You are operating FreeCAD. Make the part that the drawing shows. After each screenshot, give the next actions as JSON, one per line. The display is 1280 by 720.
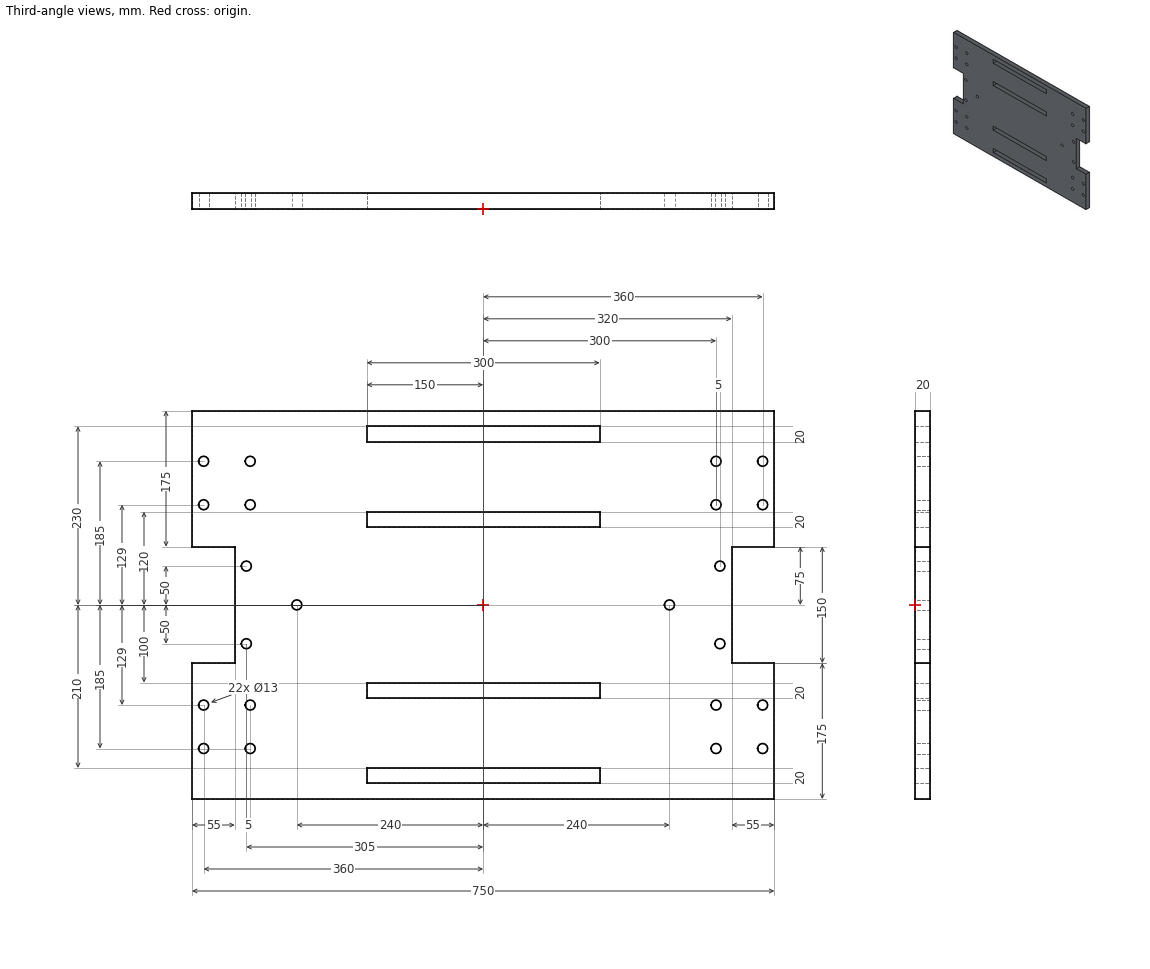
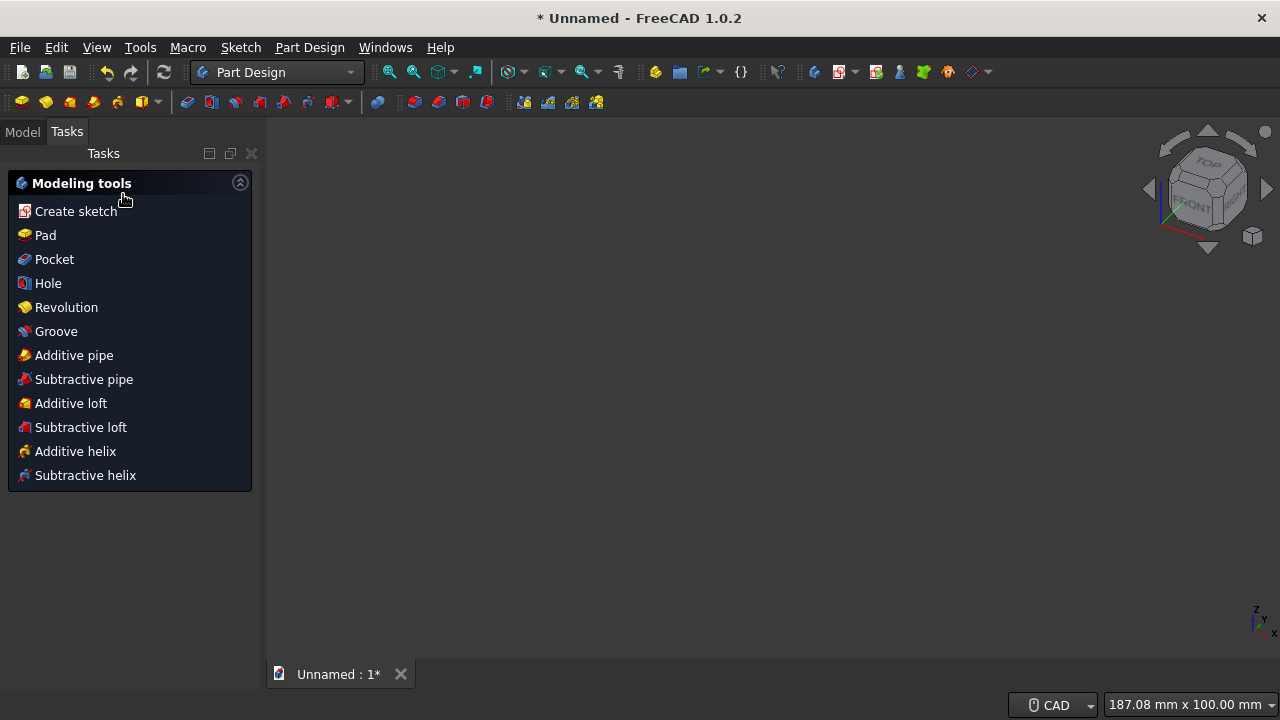
{"action": "left_click", "coordinate": [22, 102]}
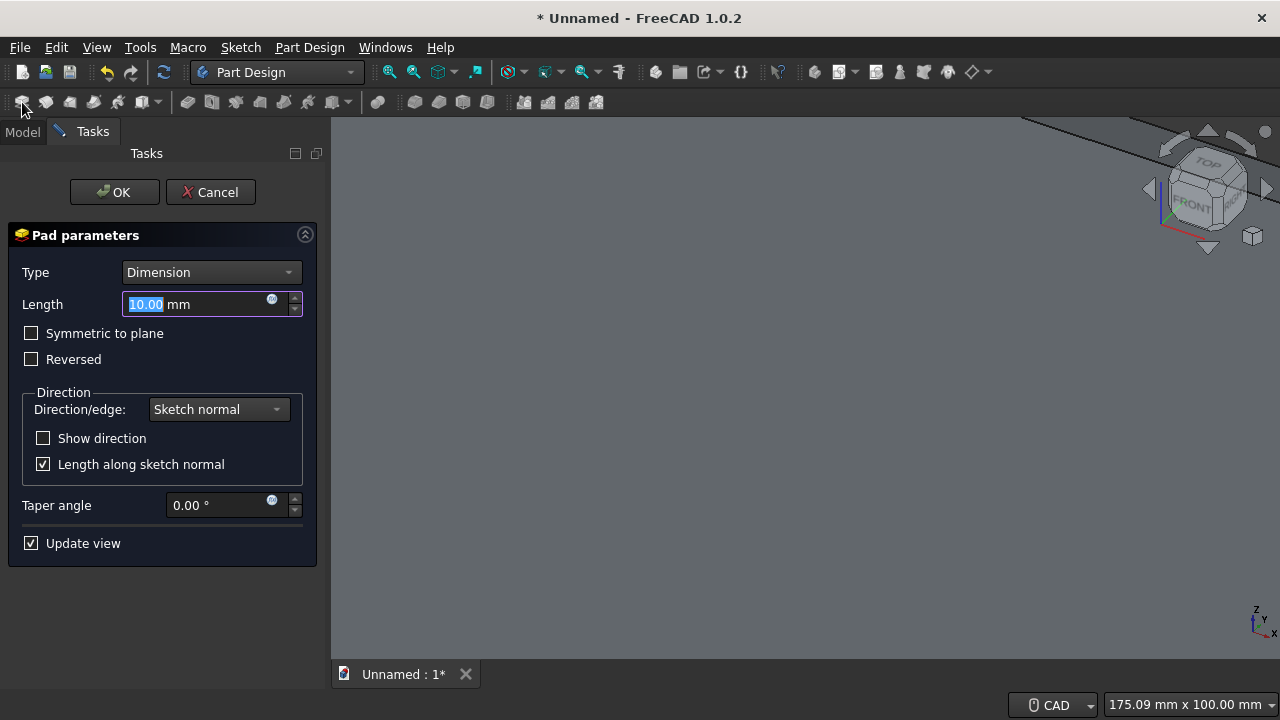
{"action": "type", "text": "20"}
{"action": "key", "text": "Tab"}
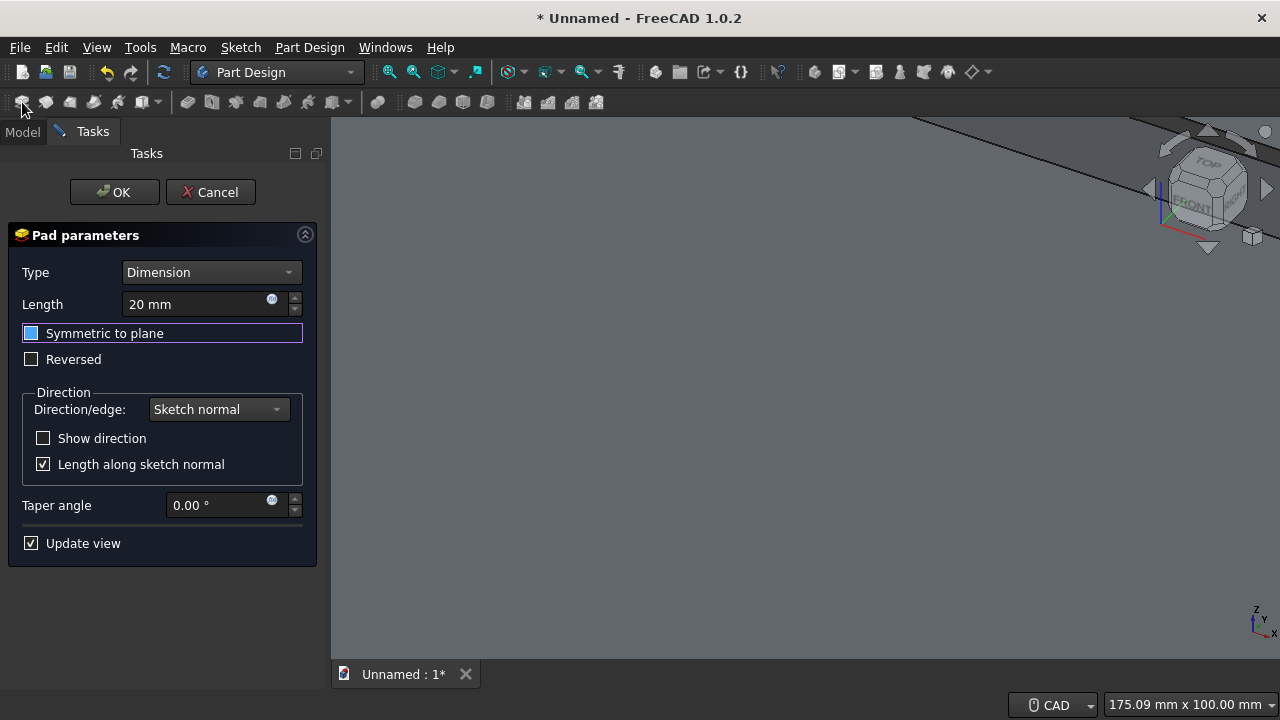
{"action": "left_click", "coordinate": [30, 359]}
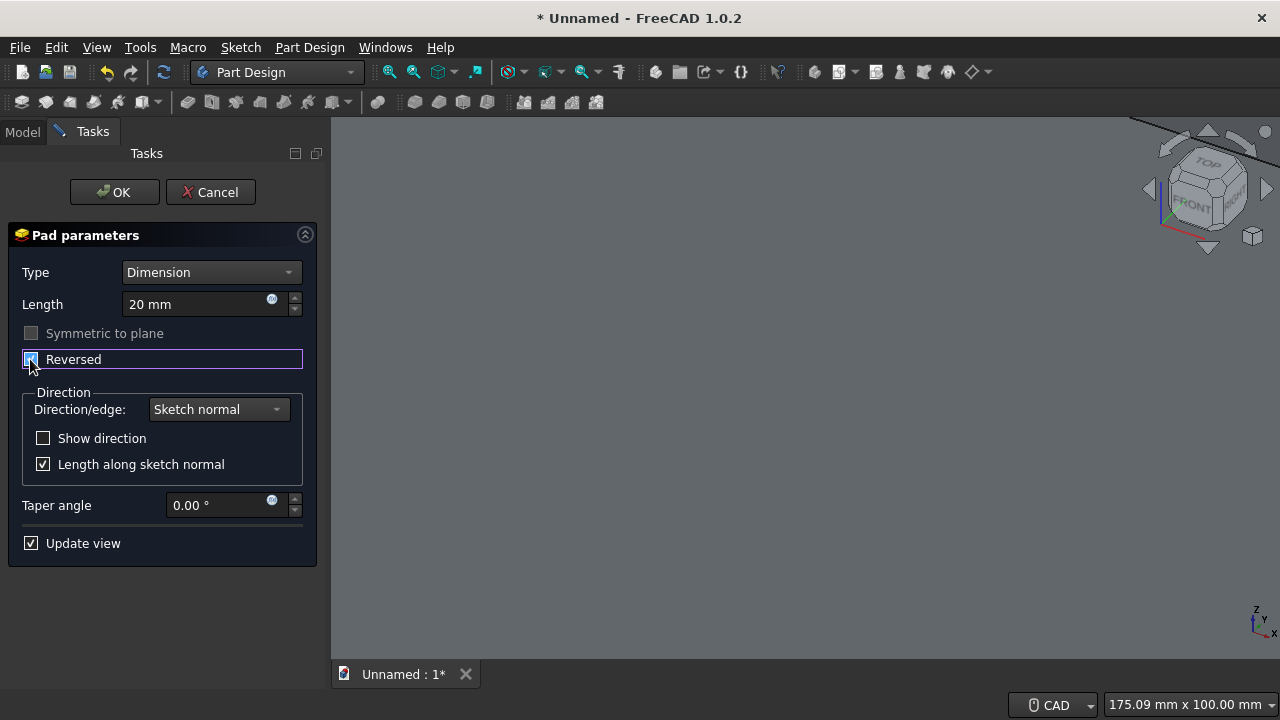
{"action": "left_click", "coordinate": [115, 192]}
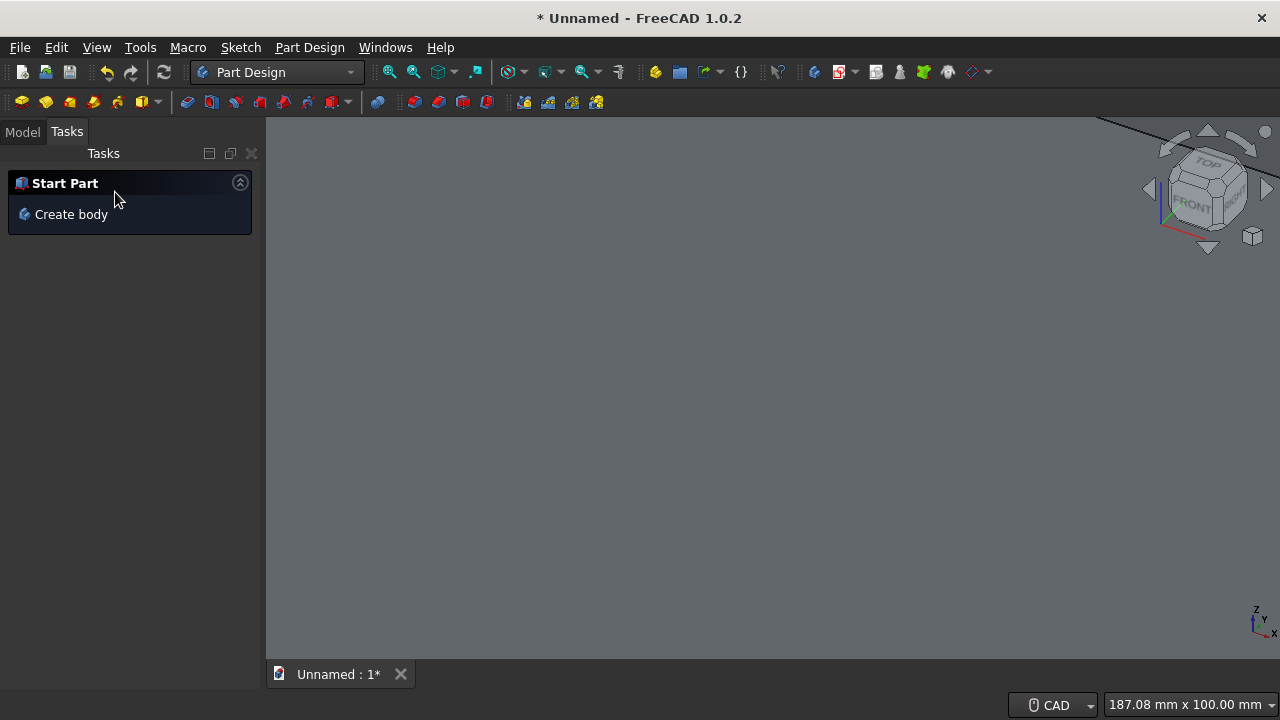
{"action": "left_click", "coordinate": [390, 72]}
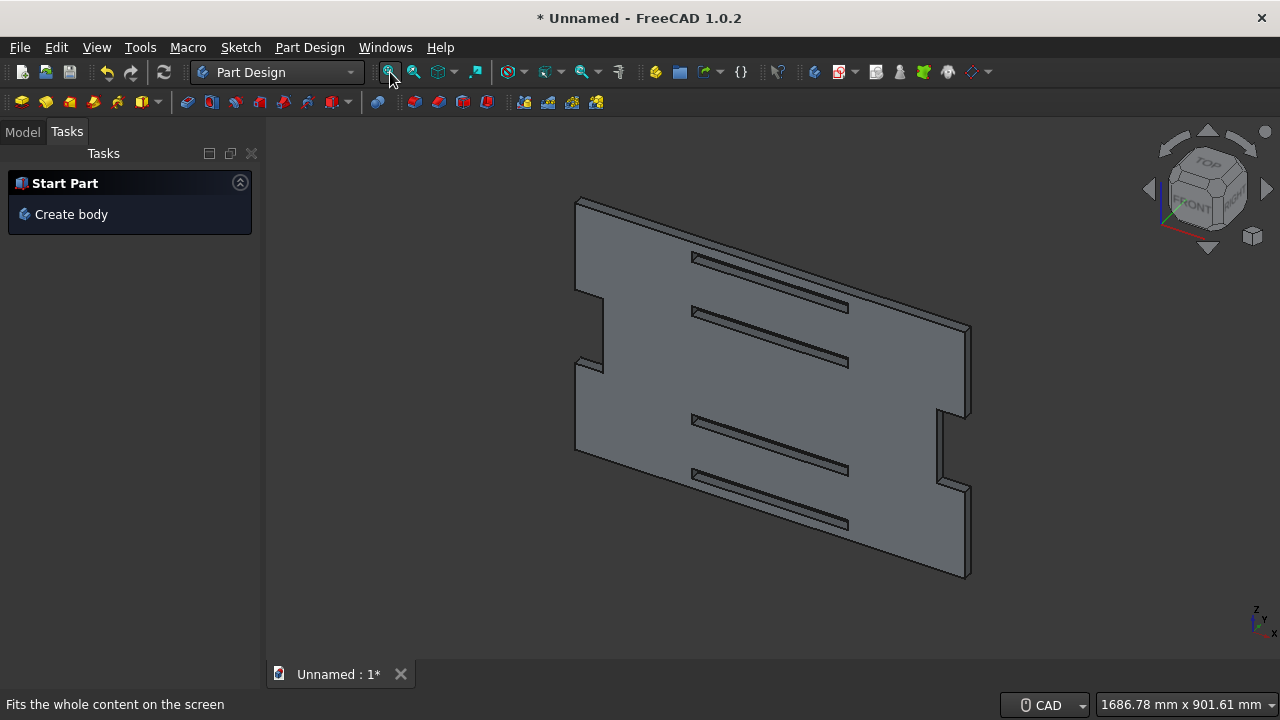
{"action": "key", "text": "4"}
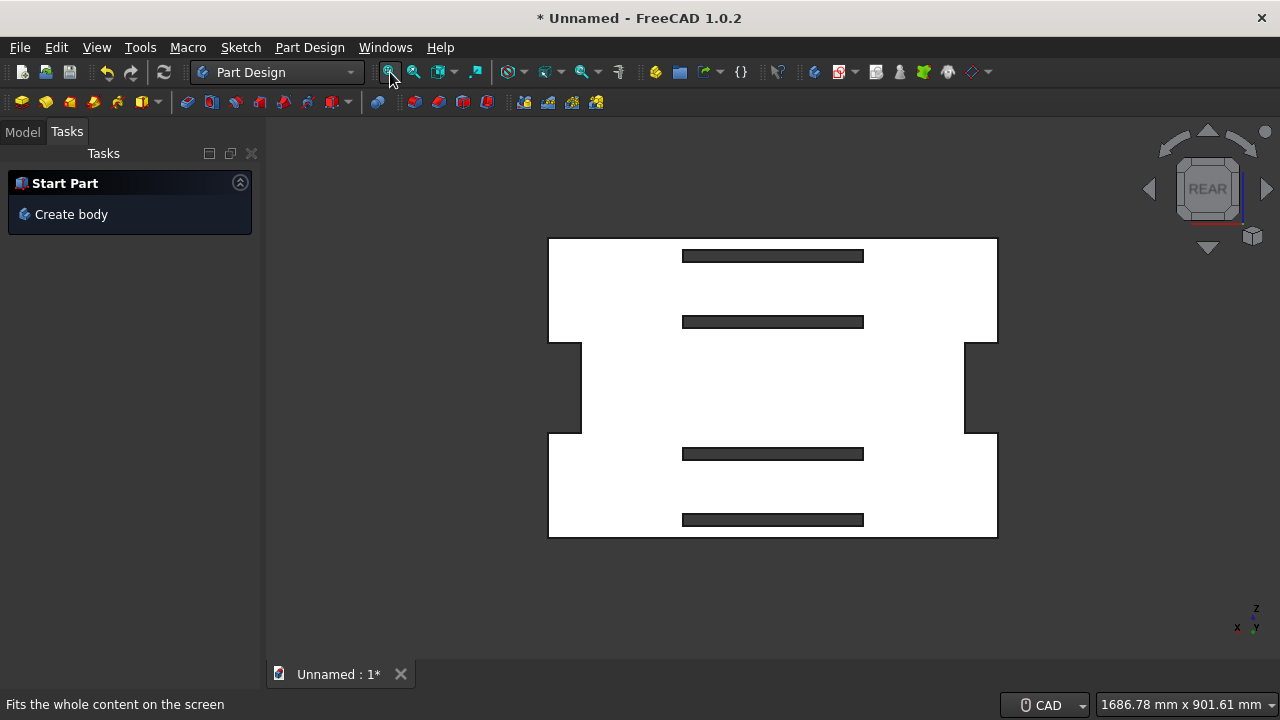
{"action": "left_click", "coordinate": [644, 387]}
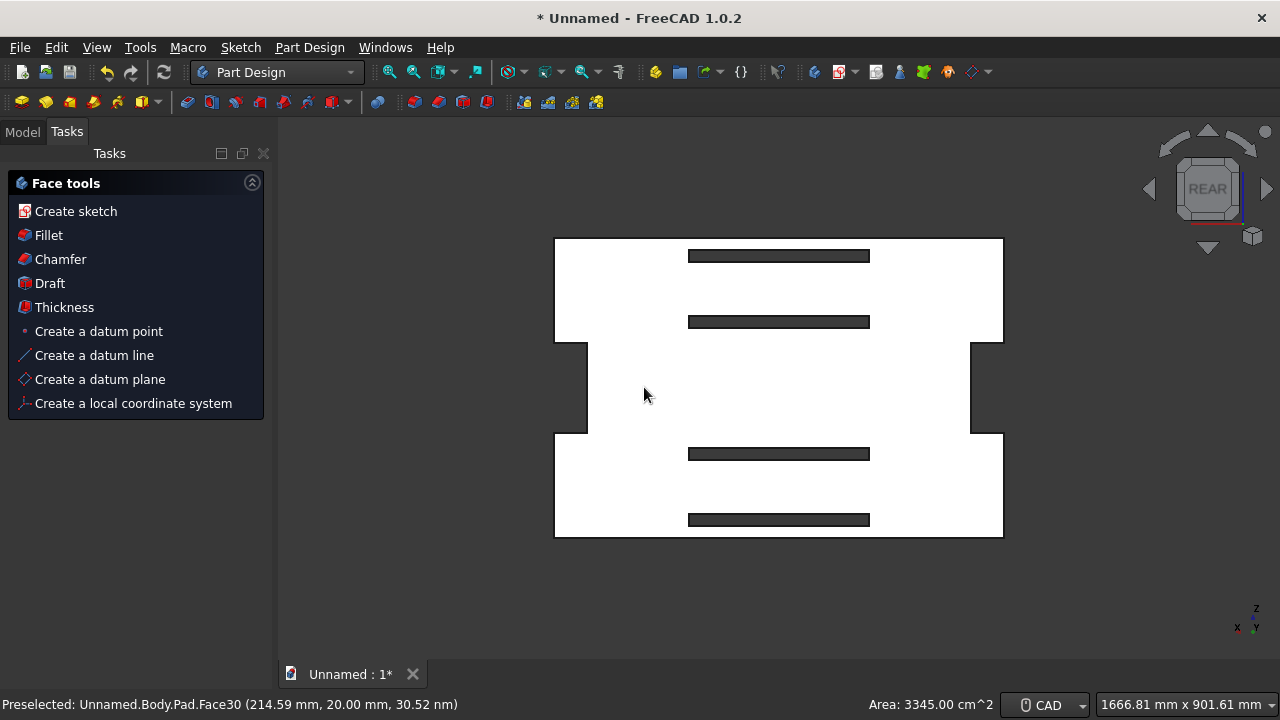
{"action": "left_click", "coordinate": [840, 72]}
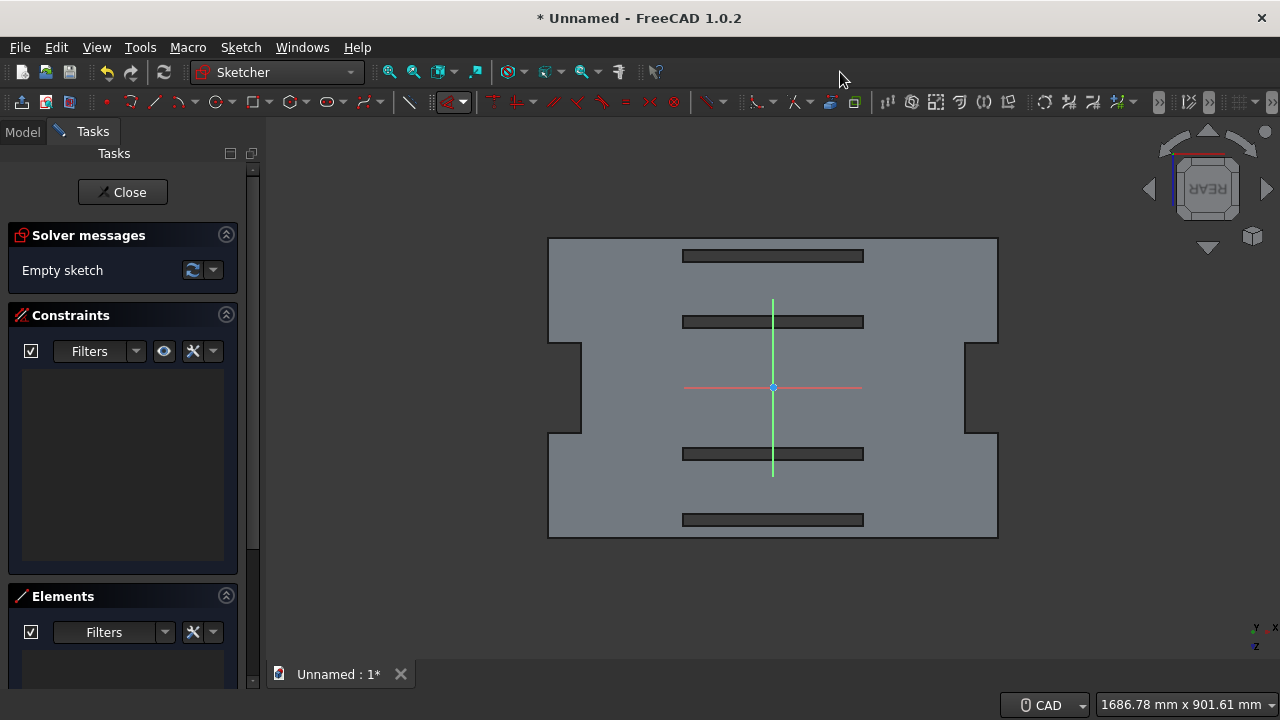
{"action": "left_click", "coordinate": [216, 102]}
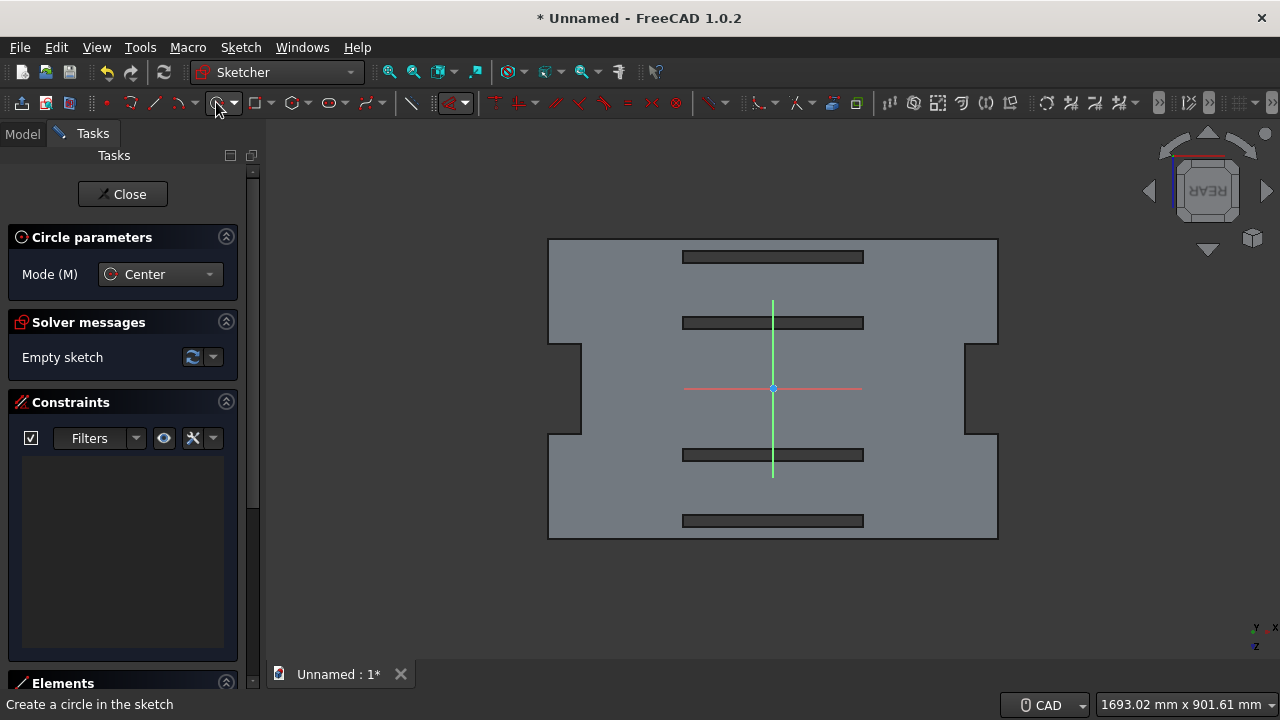
{"action": "scroll", "coordinate": [557, 312], "scroll_direction": "up", "scroll_amount": 9}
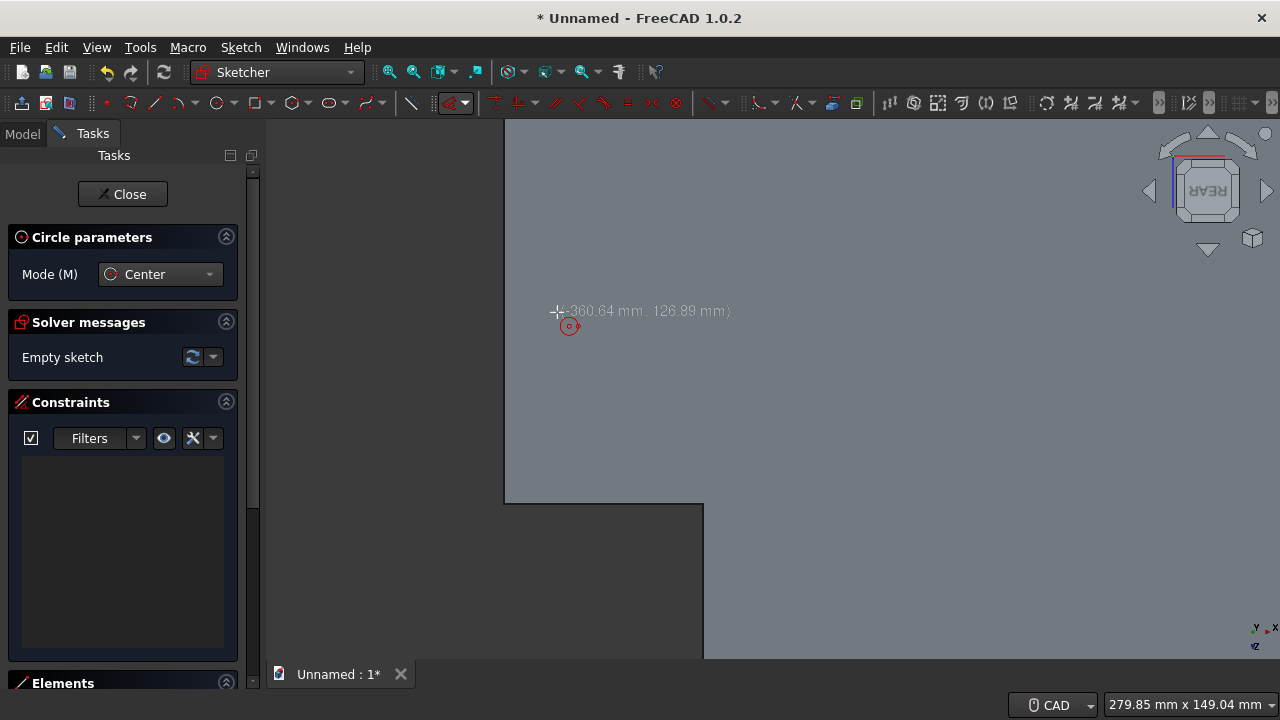
{"action": "scroll", "coordinate": [412, 291], "scroll_direction": "down", "scroll_amount": 8}